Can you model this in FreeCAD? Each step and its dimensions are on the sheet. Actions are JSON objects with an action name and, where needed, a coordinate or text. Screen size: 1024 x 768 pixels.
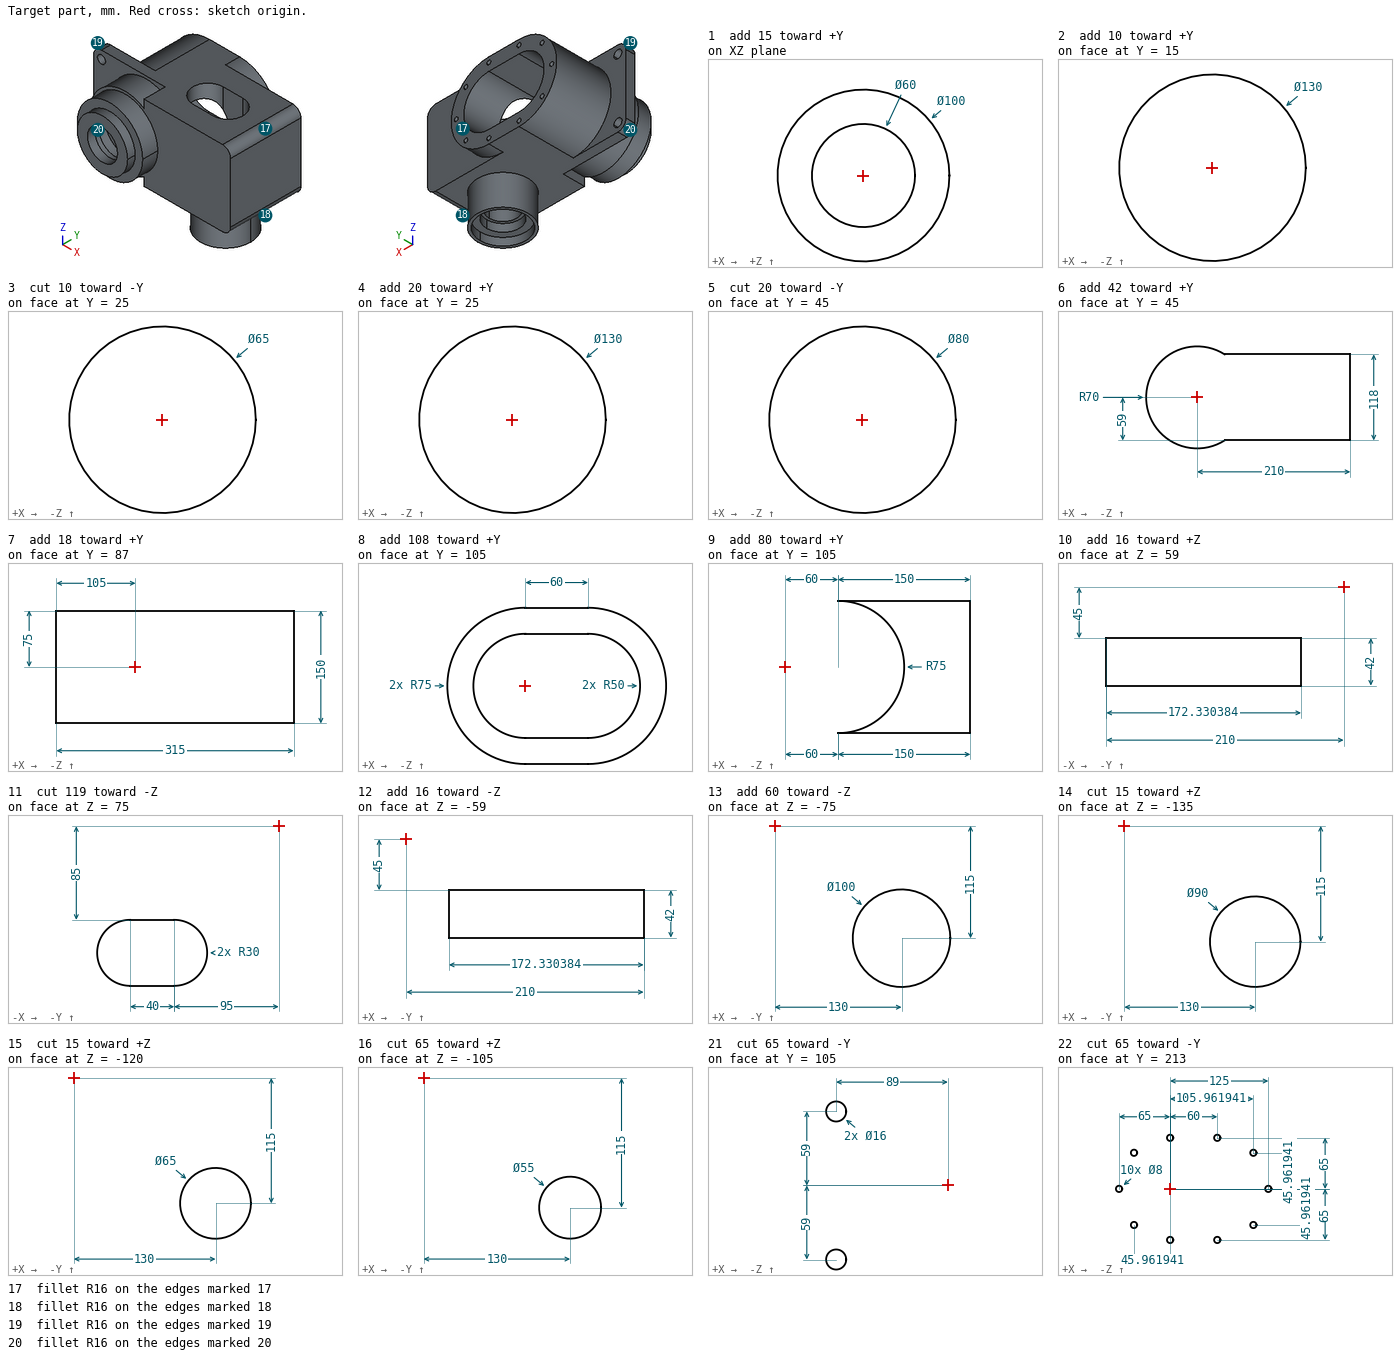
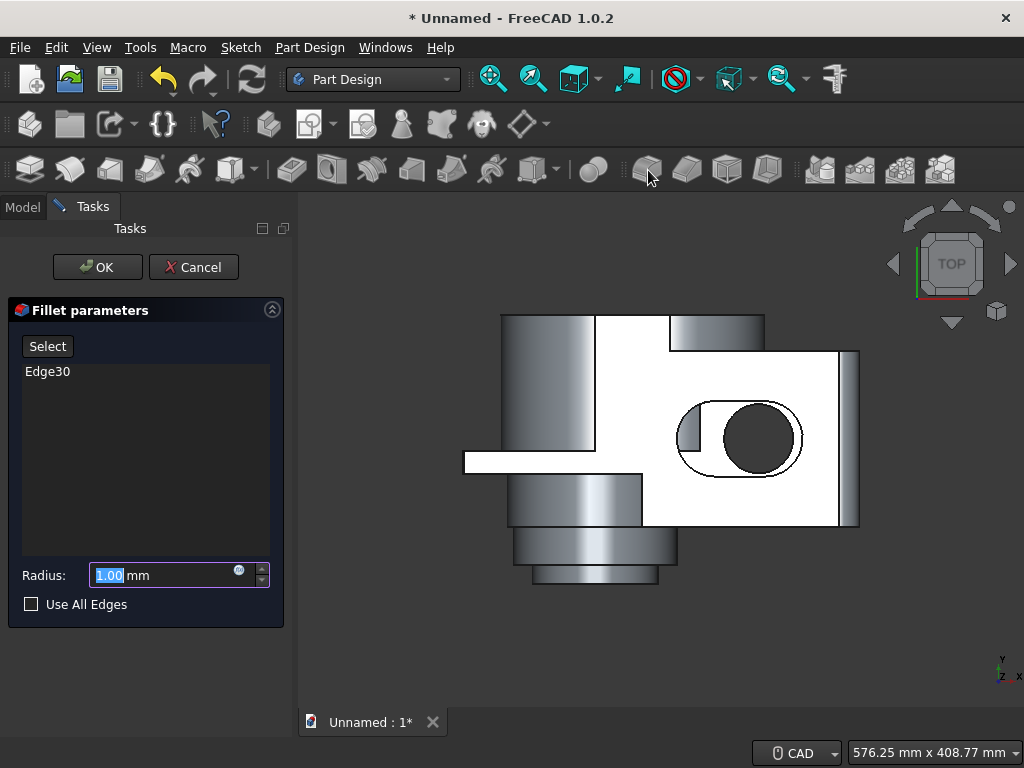
{"action": "type", "text": "16"}
{"action": "key", "text": "Tab"}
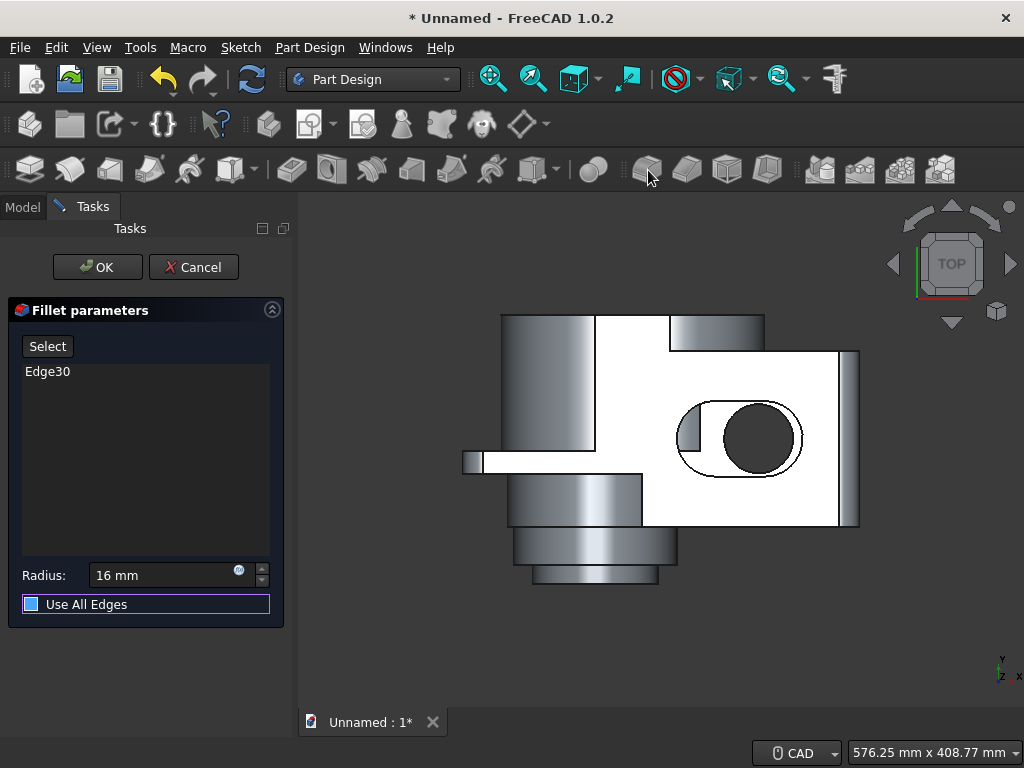
{"action": "left_click", "coordinate": [98, 267]}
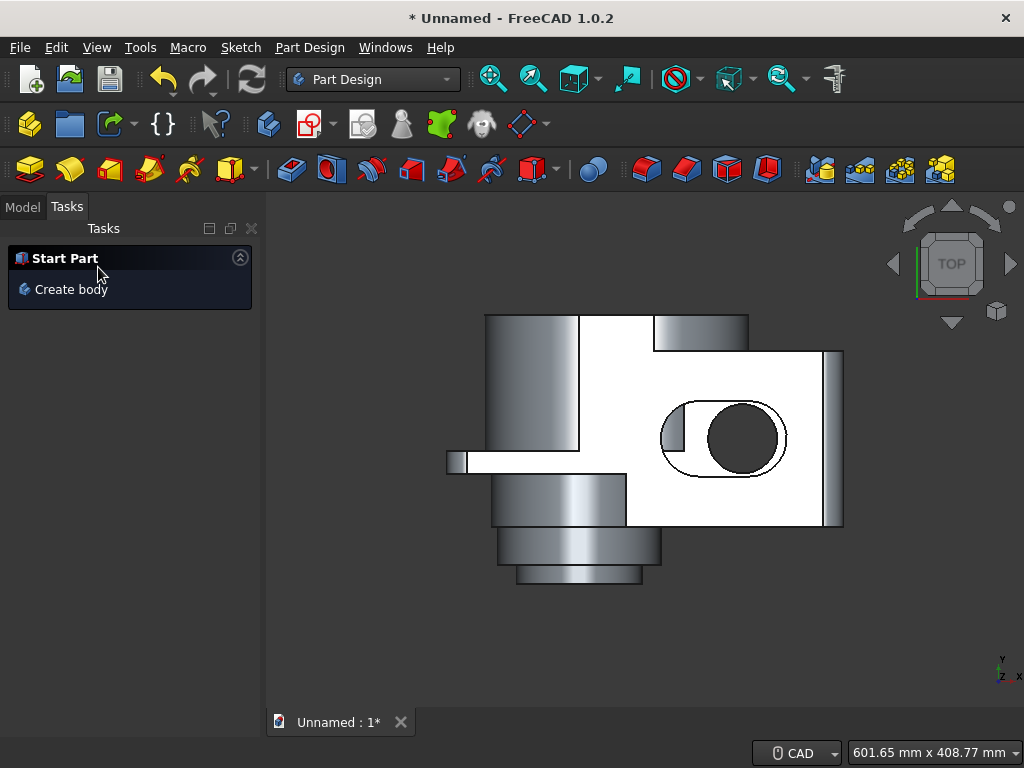
{"action": "key", "text": "0"}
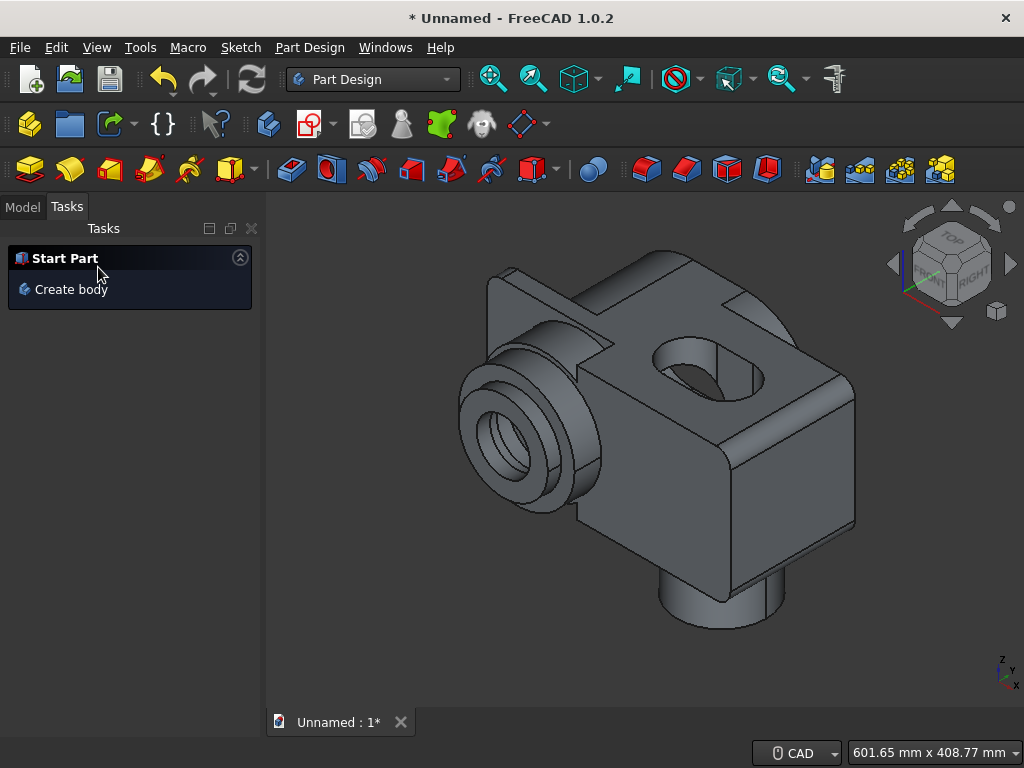
{"action": "key", "text": "2"}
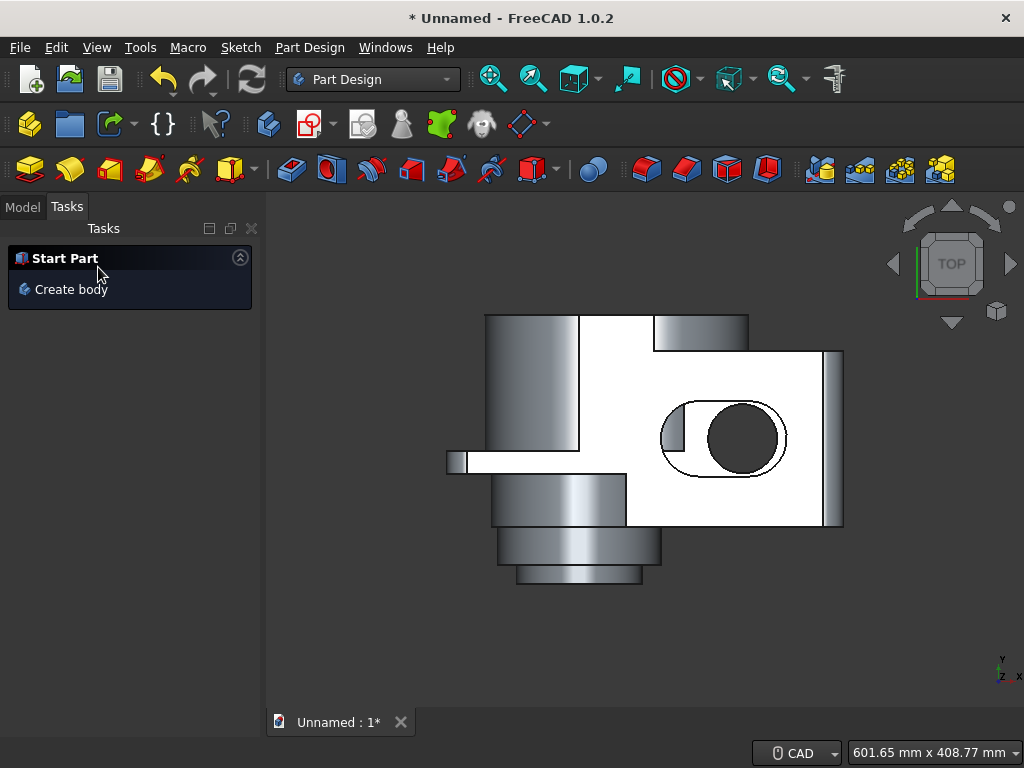
{"action": "key", "text": "1"}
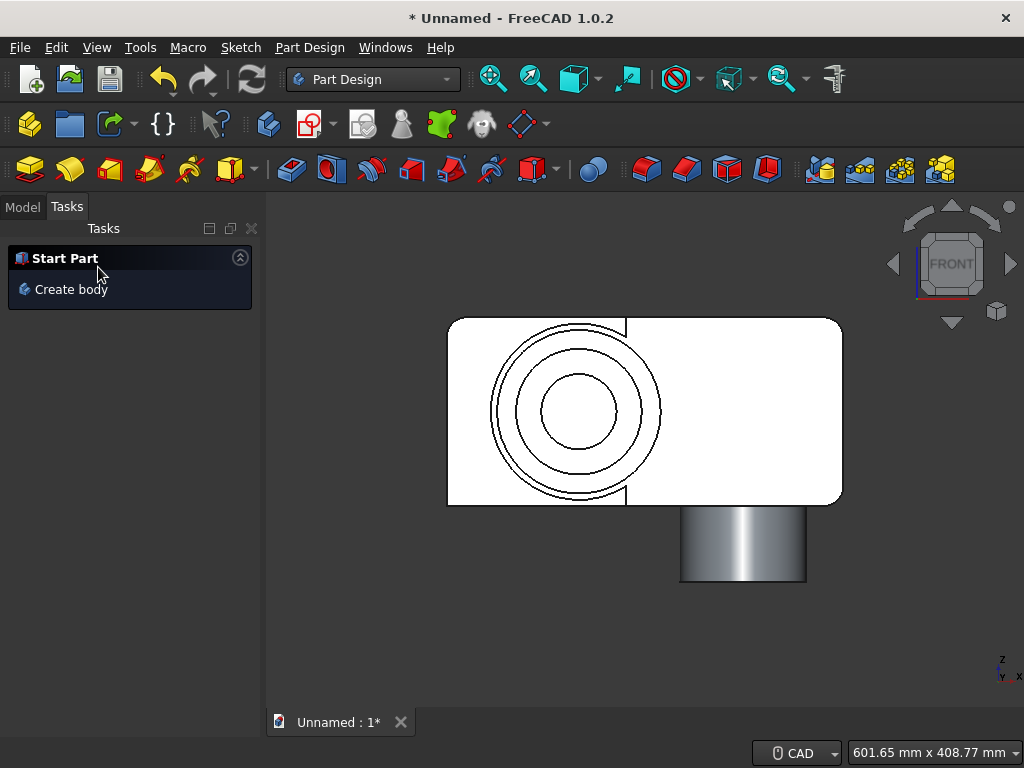
{"action": "key", "text": "3"}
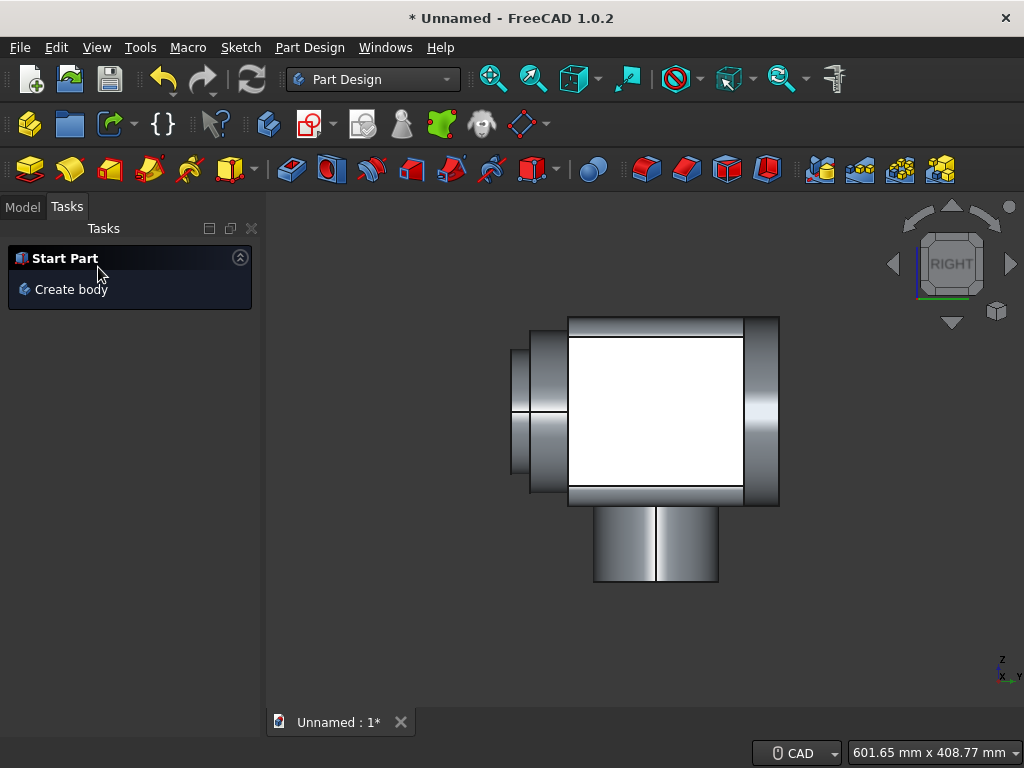
{"action": "key", "text": "5"}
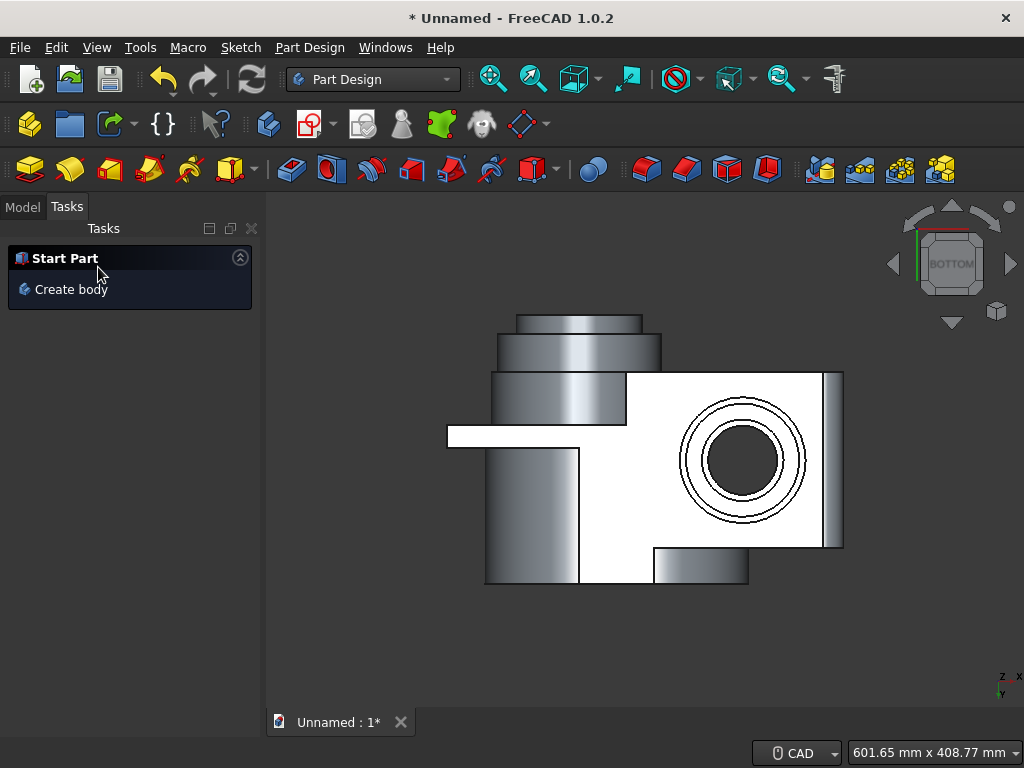
{"action": "left_click", "coordinate": [447, 435]}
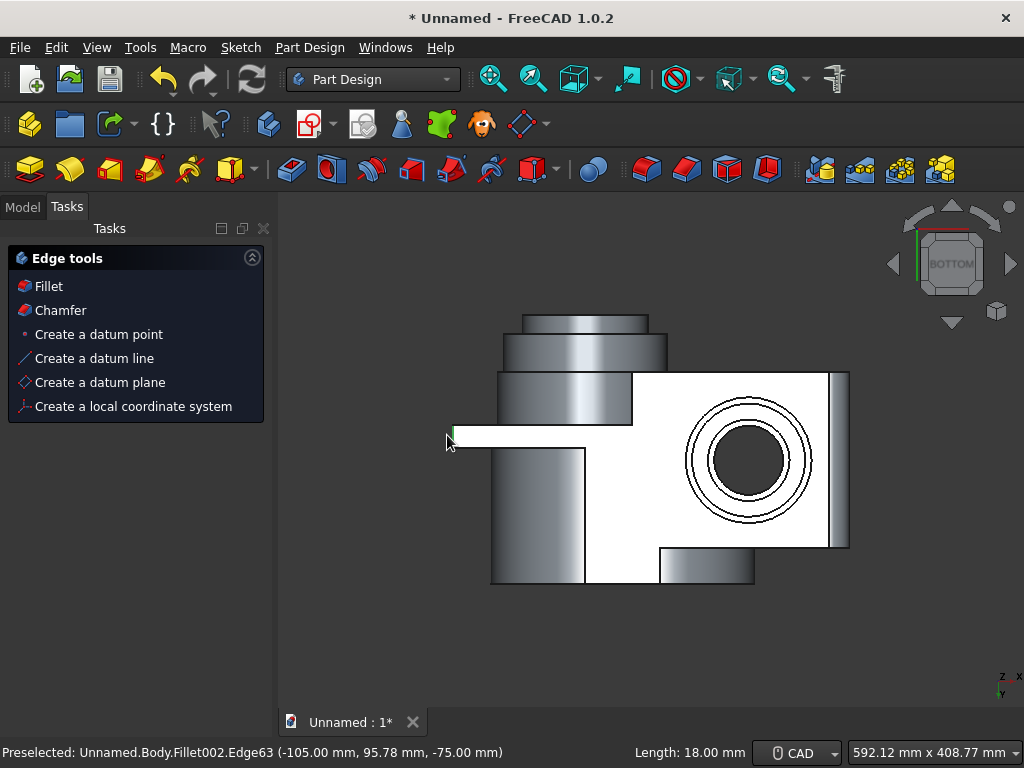
{"action": "left_click", "coordinate": [648, 170]}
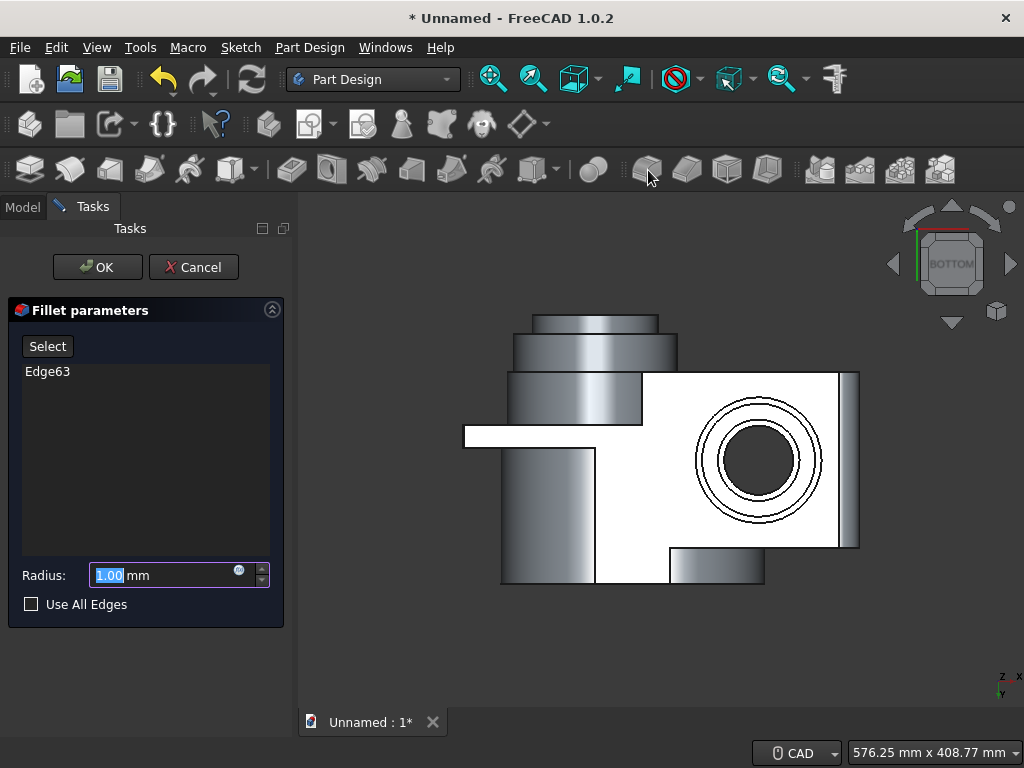
{"action": "type", "text": "16"}
{"action": "key", "text": "Tab"}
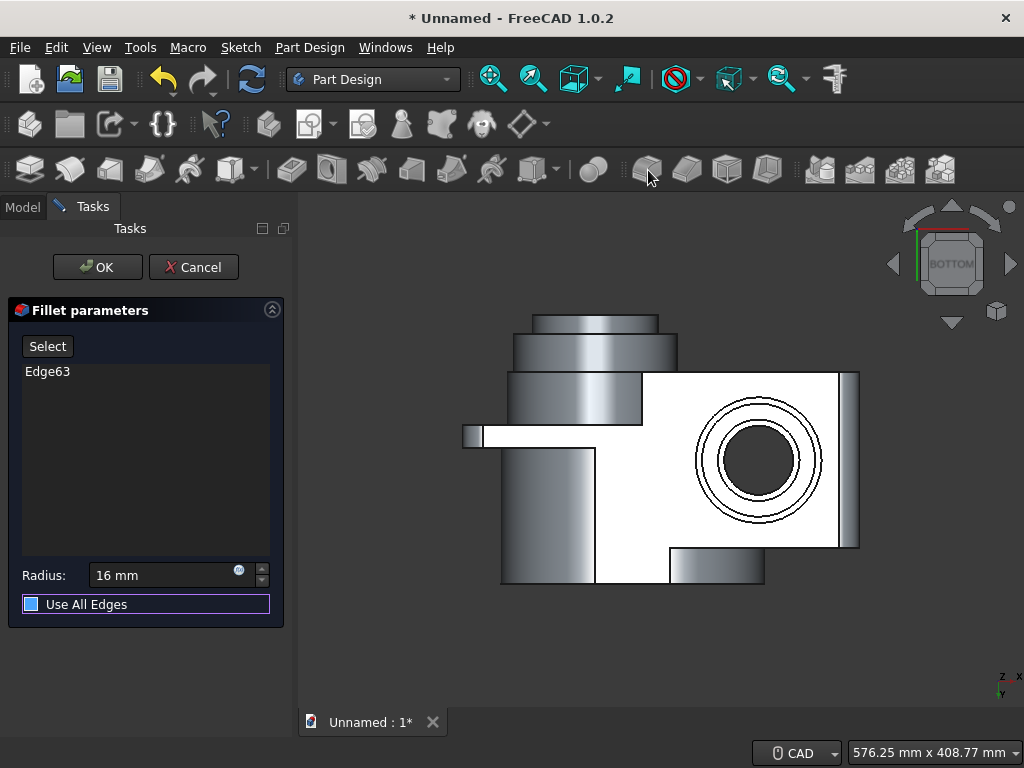
{"action": "left_click", "coordinate": [98, 267]}